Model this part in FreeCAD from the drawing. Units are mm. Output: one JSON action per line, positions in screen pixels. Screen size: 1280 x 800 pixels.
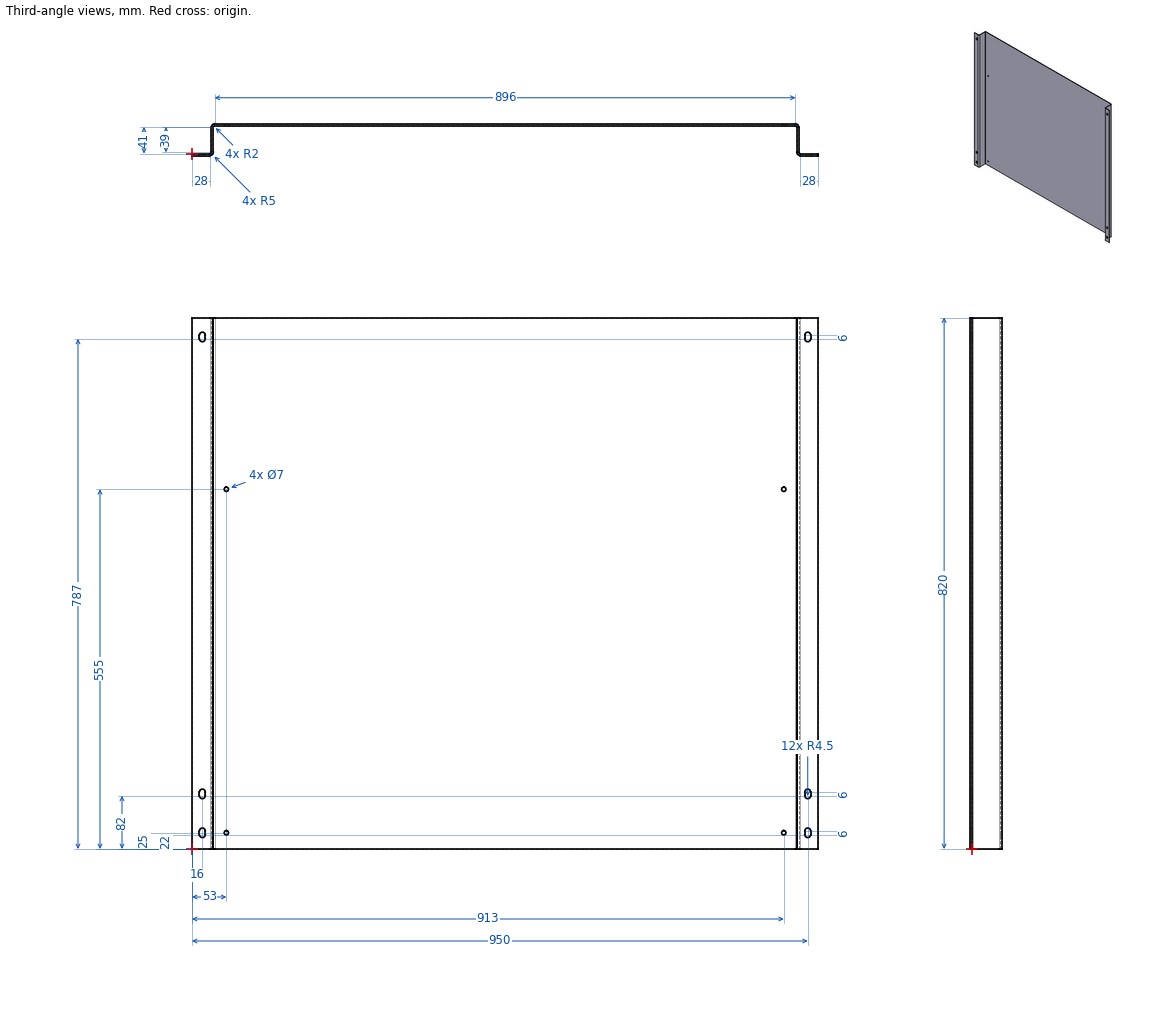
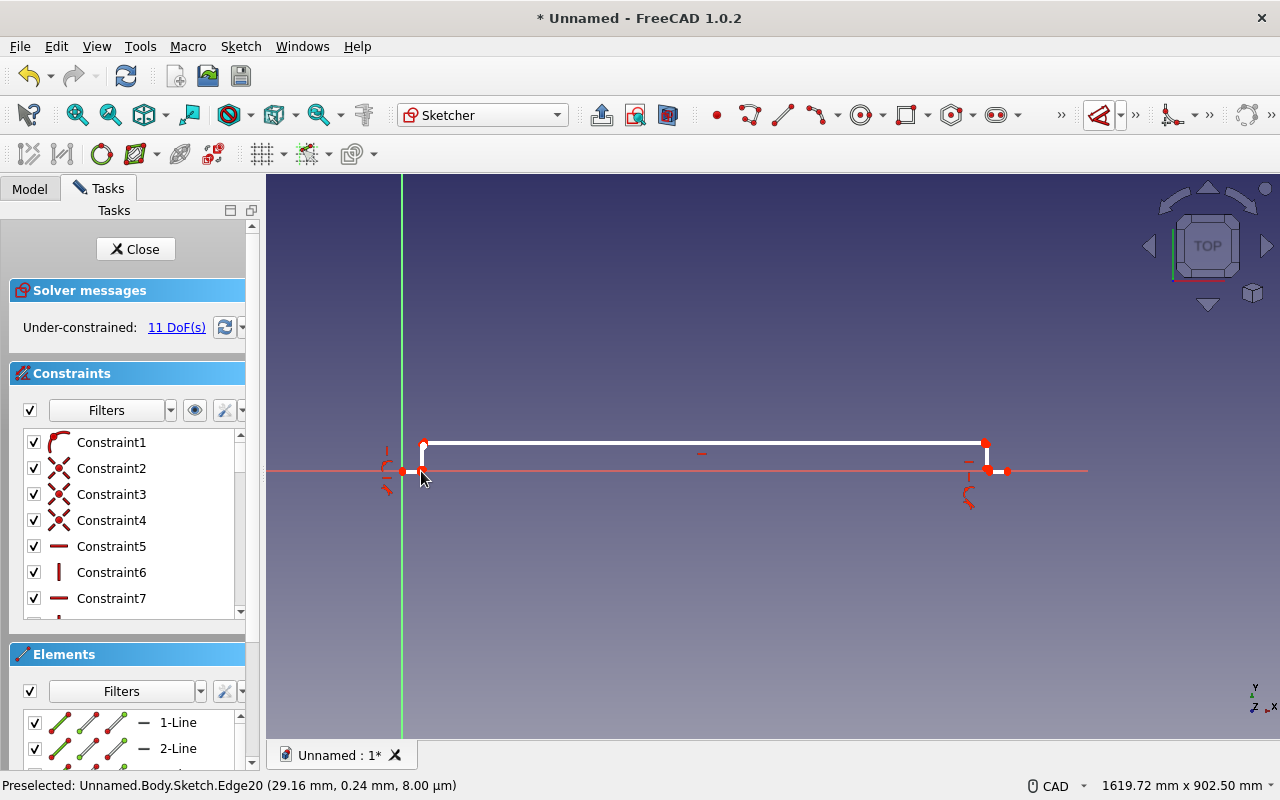
{"action": "scroll", "coordinate": [424, 444], "scroll_direction": "up", "scroll_amount": 14}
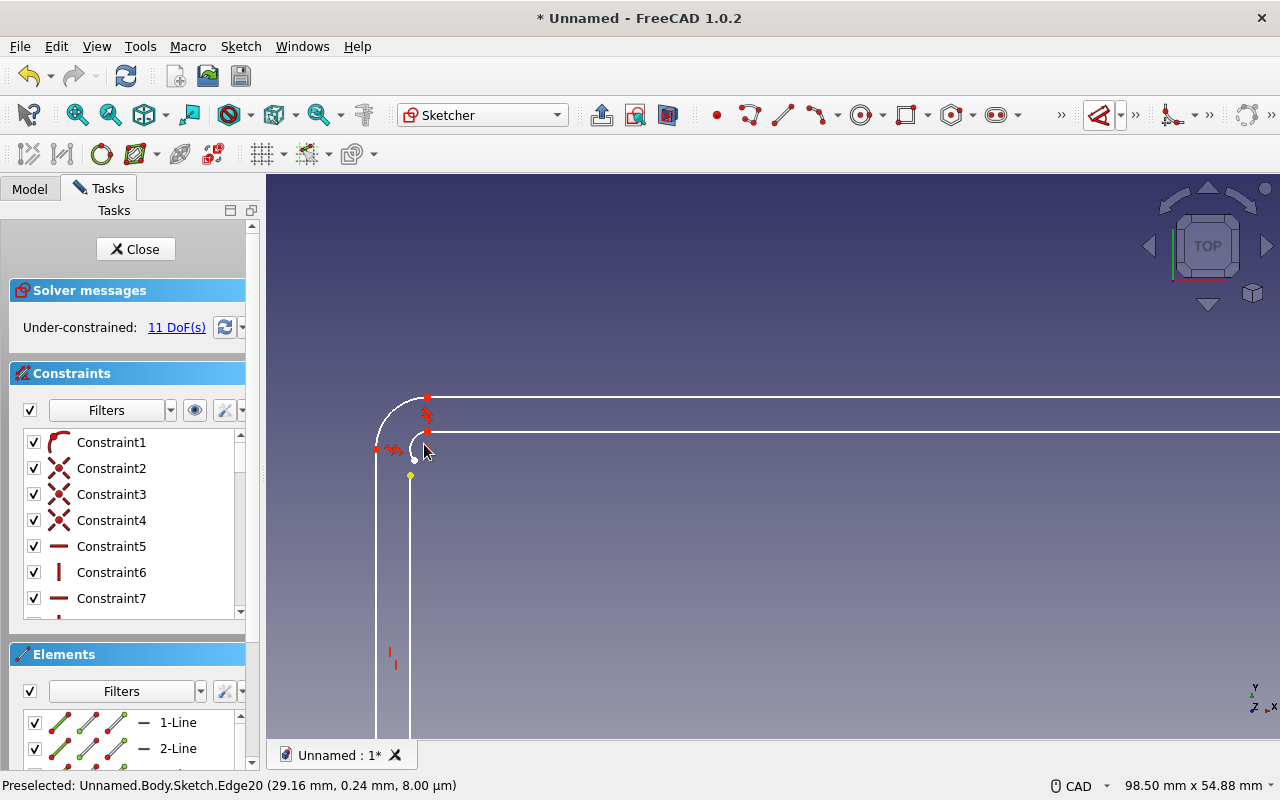
{"action": "left_click", "coordinate": [417, 435]}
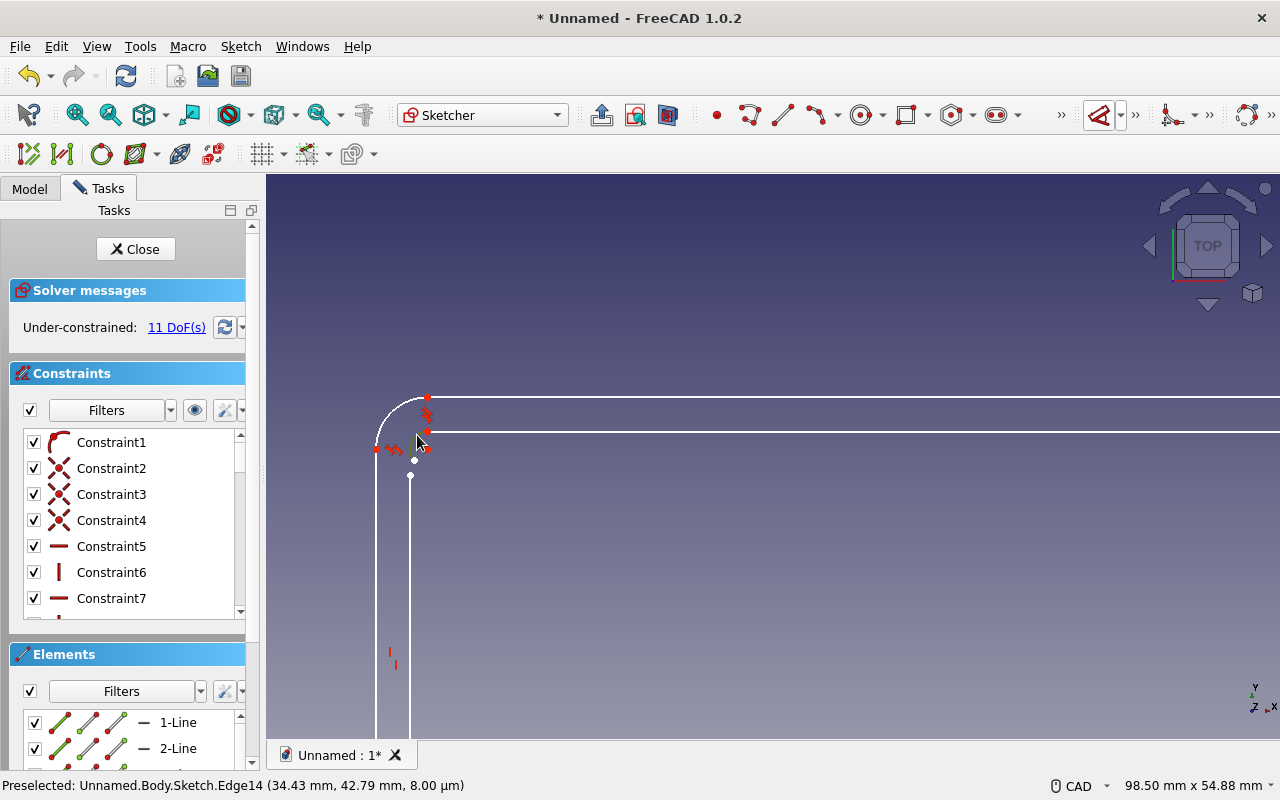
{"action": "scroll", "coordinate": [424, 444], "scroll_direction": "down", "scroll_amount": 14}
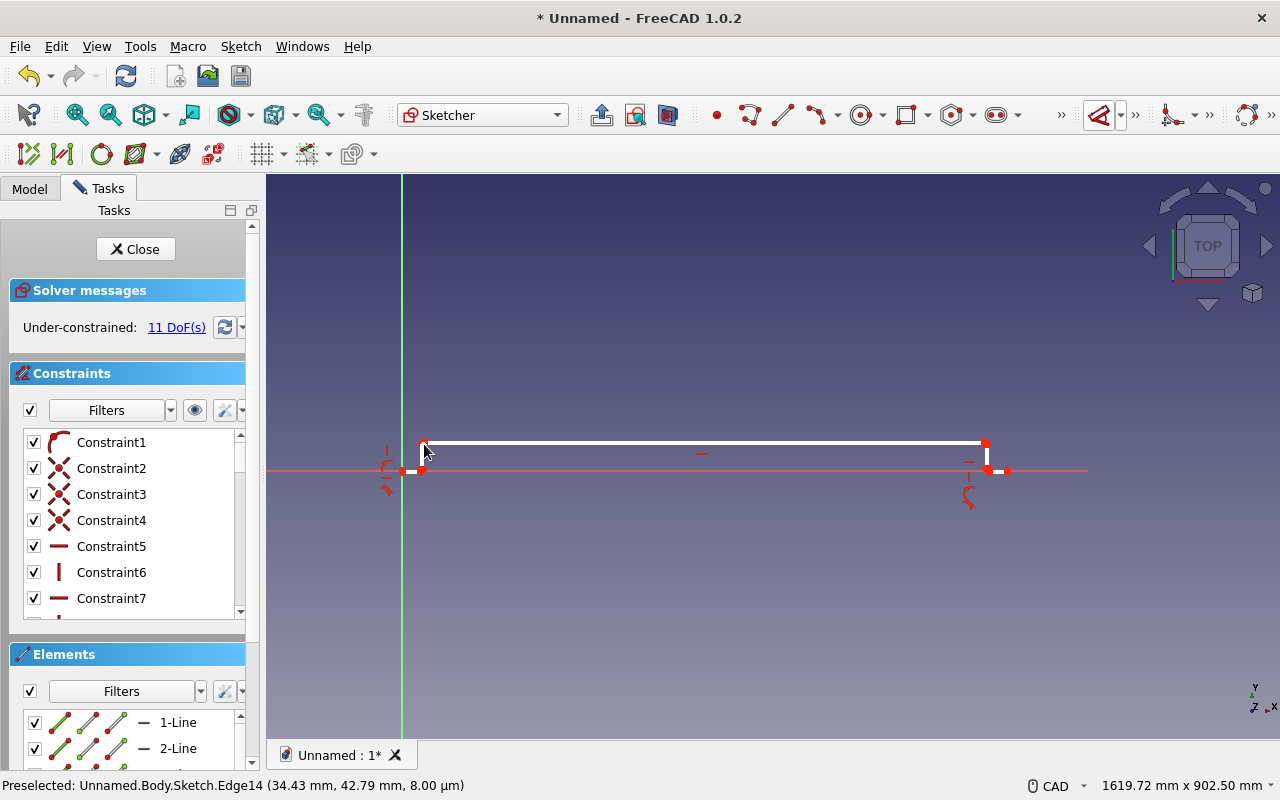
{"action": "scroll", "coordinate": [986, 444], "scroll_direction": "up", "scroll_amount": 14}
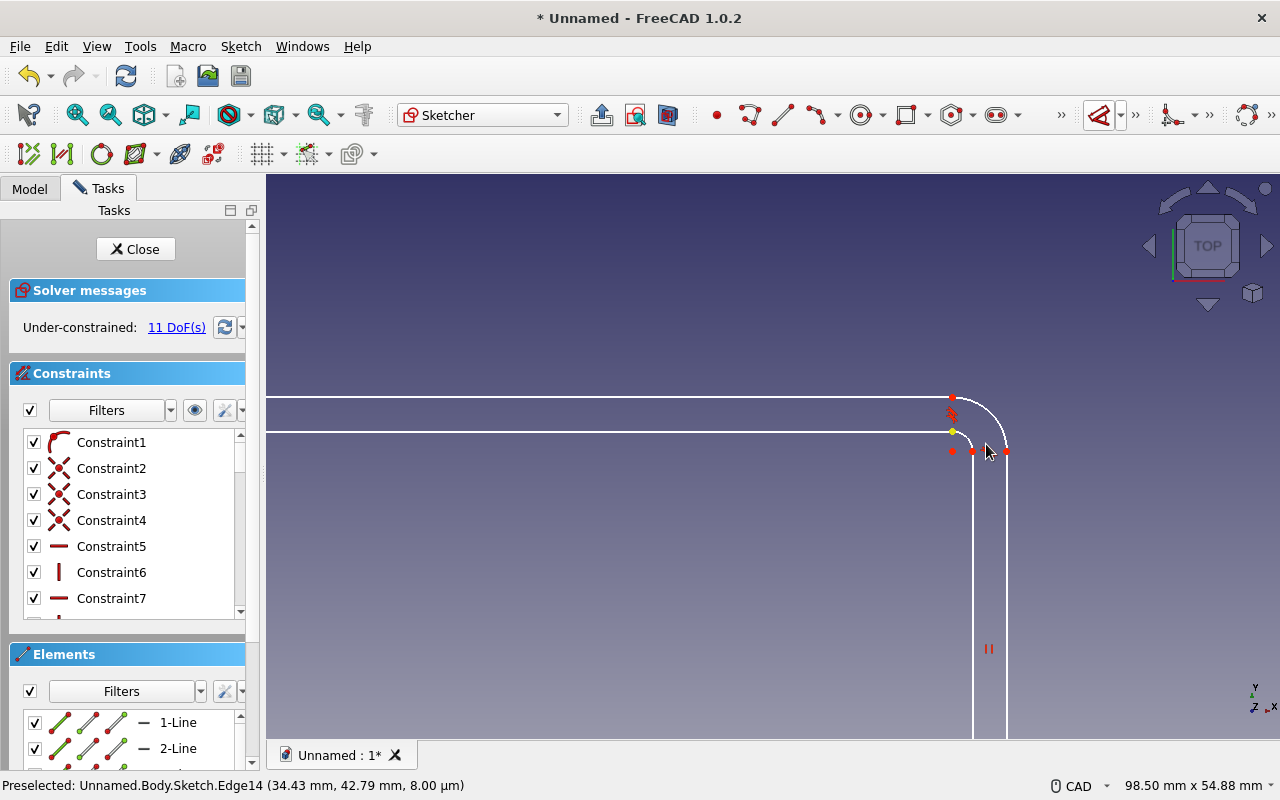
{"action": "left_click", "coordinate": [971, 443]}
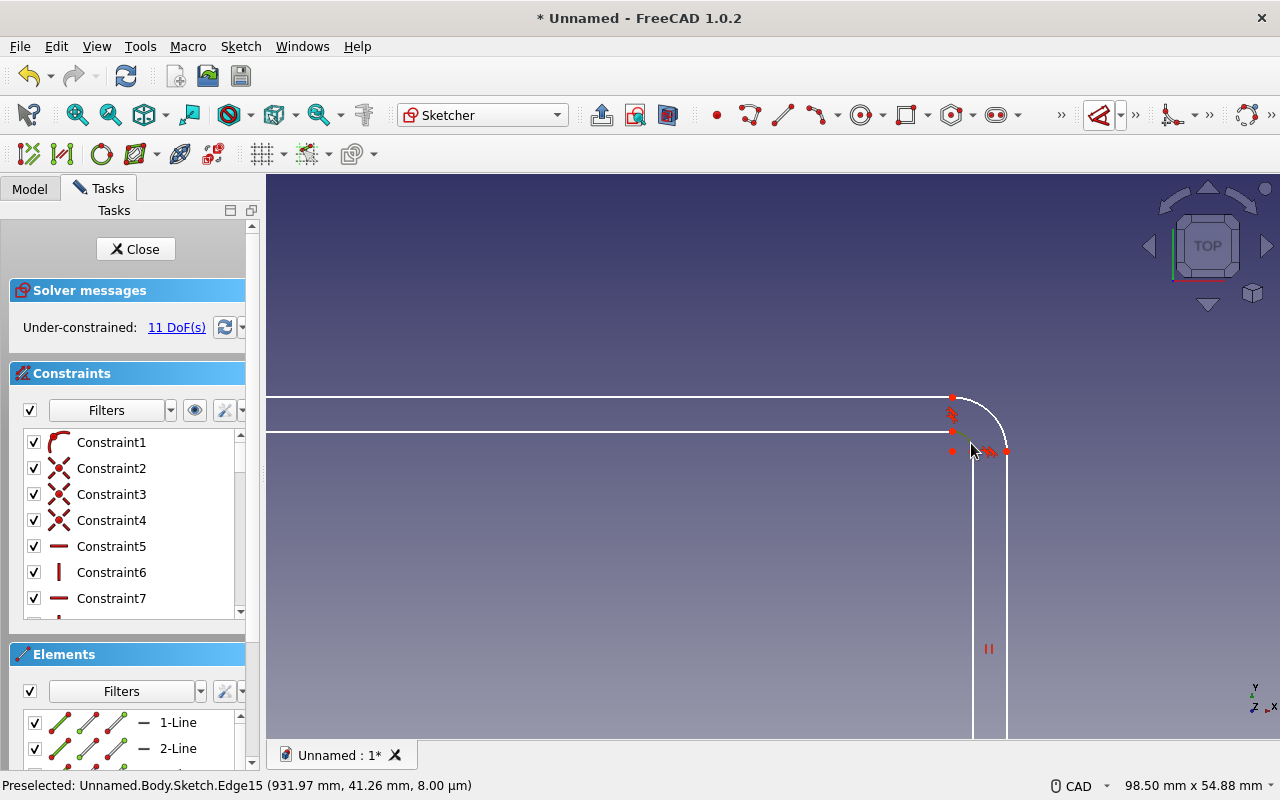
{"action": "scroll", "coordinate": [986, 444], "scroll_direction": "down", "scroll_amount": 14}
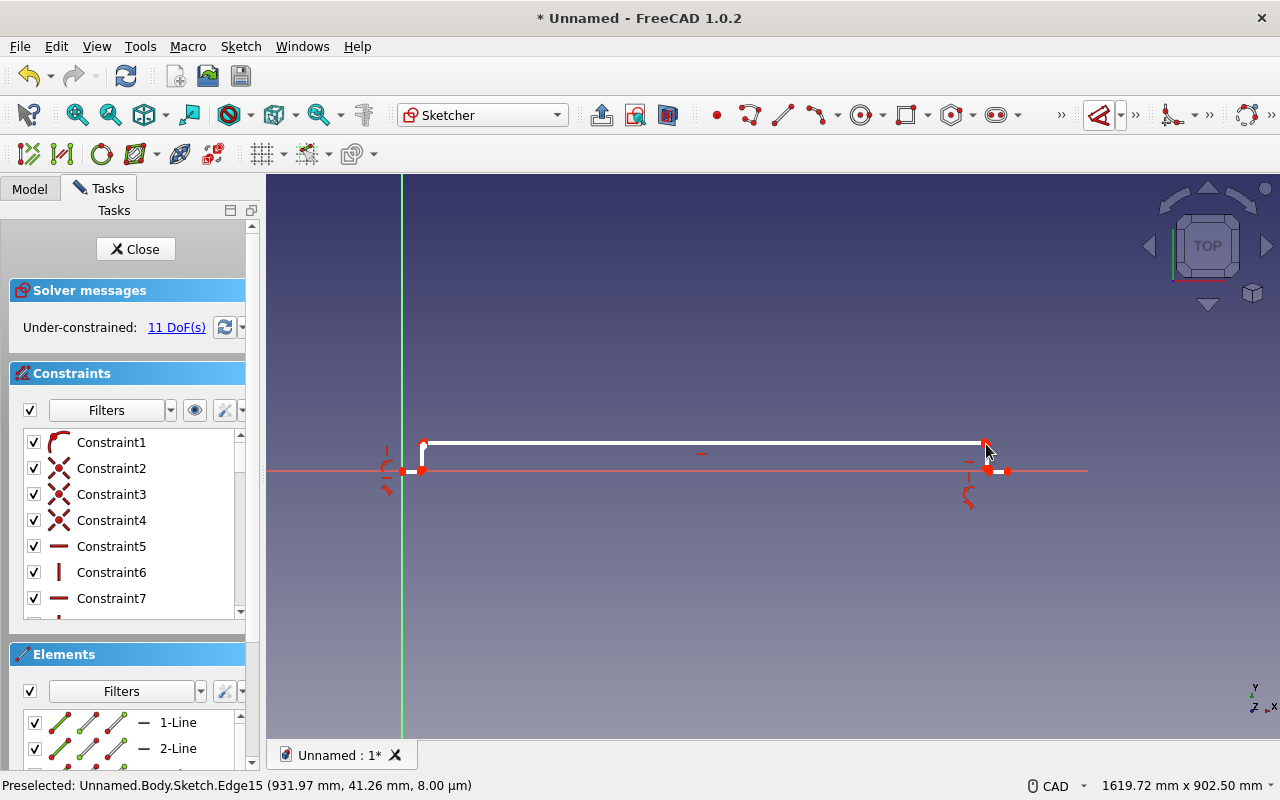
{"action": "scroll", "coordinate": [988, 470], "scroll_direction": "up", "scroll_amount": 14}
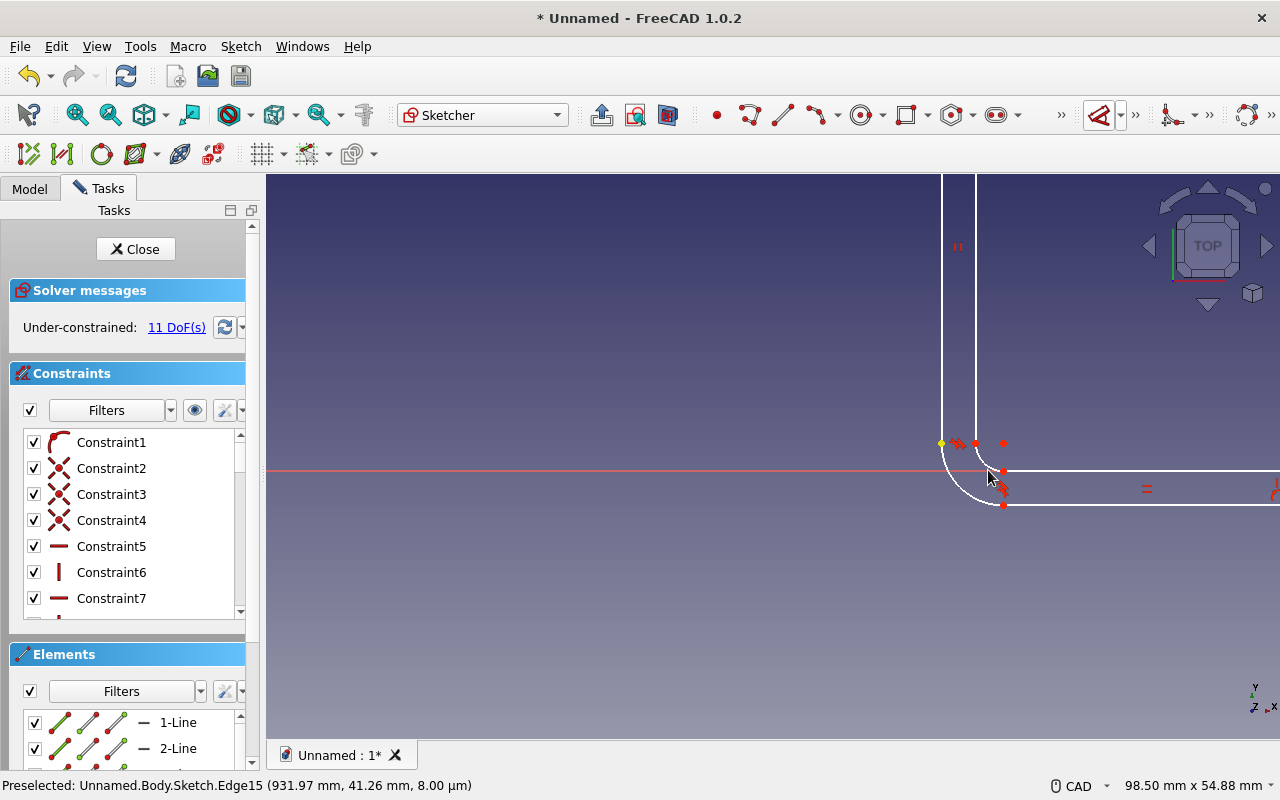
{"action": "left_click", "coordinate": [979, 456]}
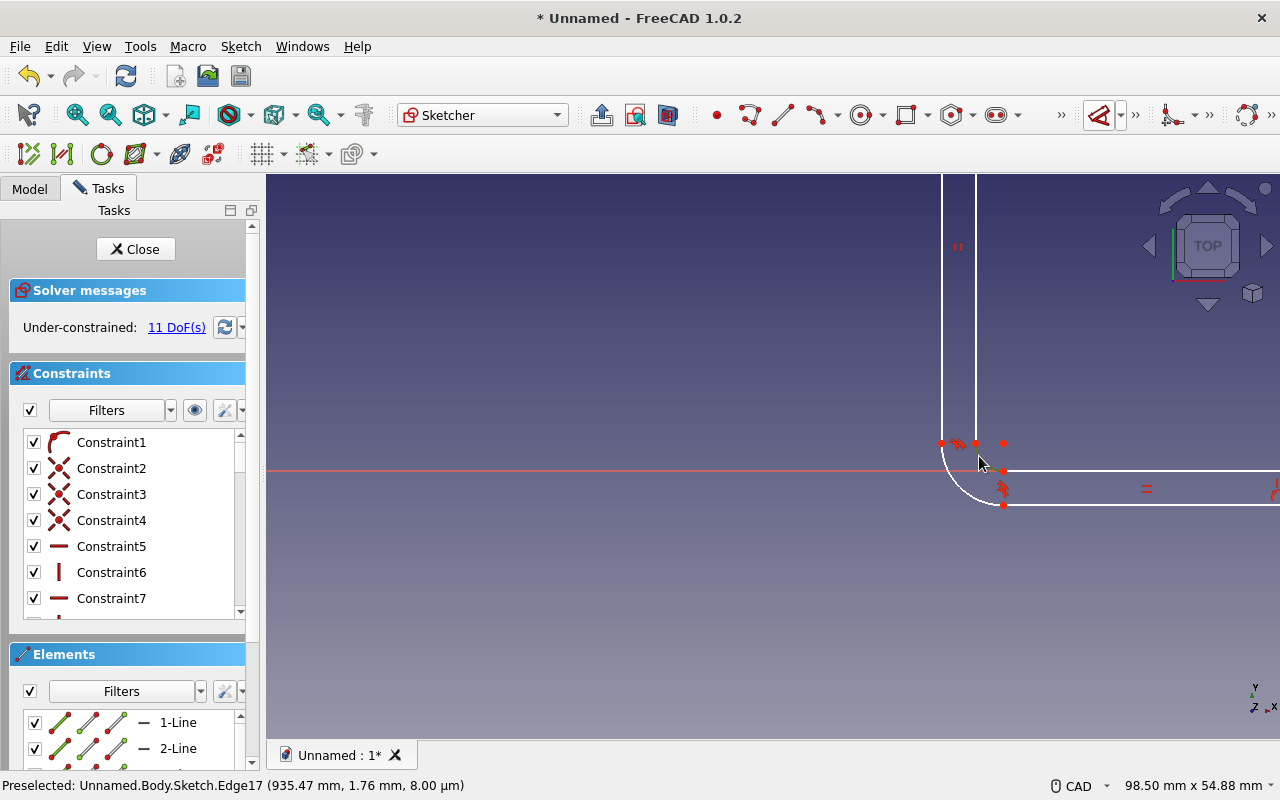
{"action": "scroll", "coordinate": [988, 470], "scroll_direction": "down", "scroll_amount": 14}